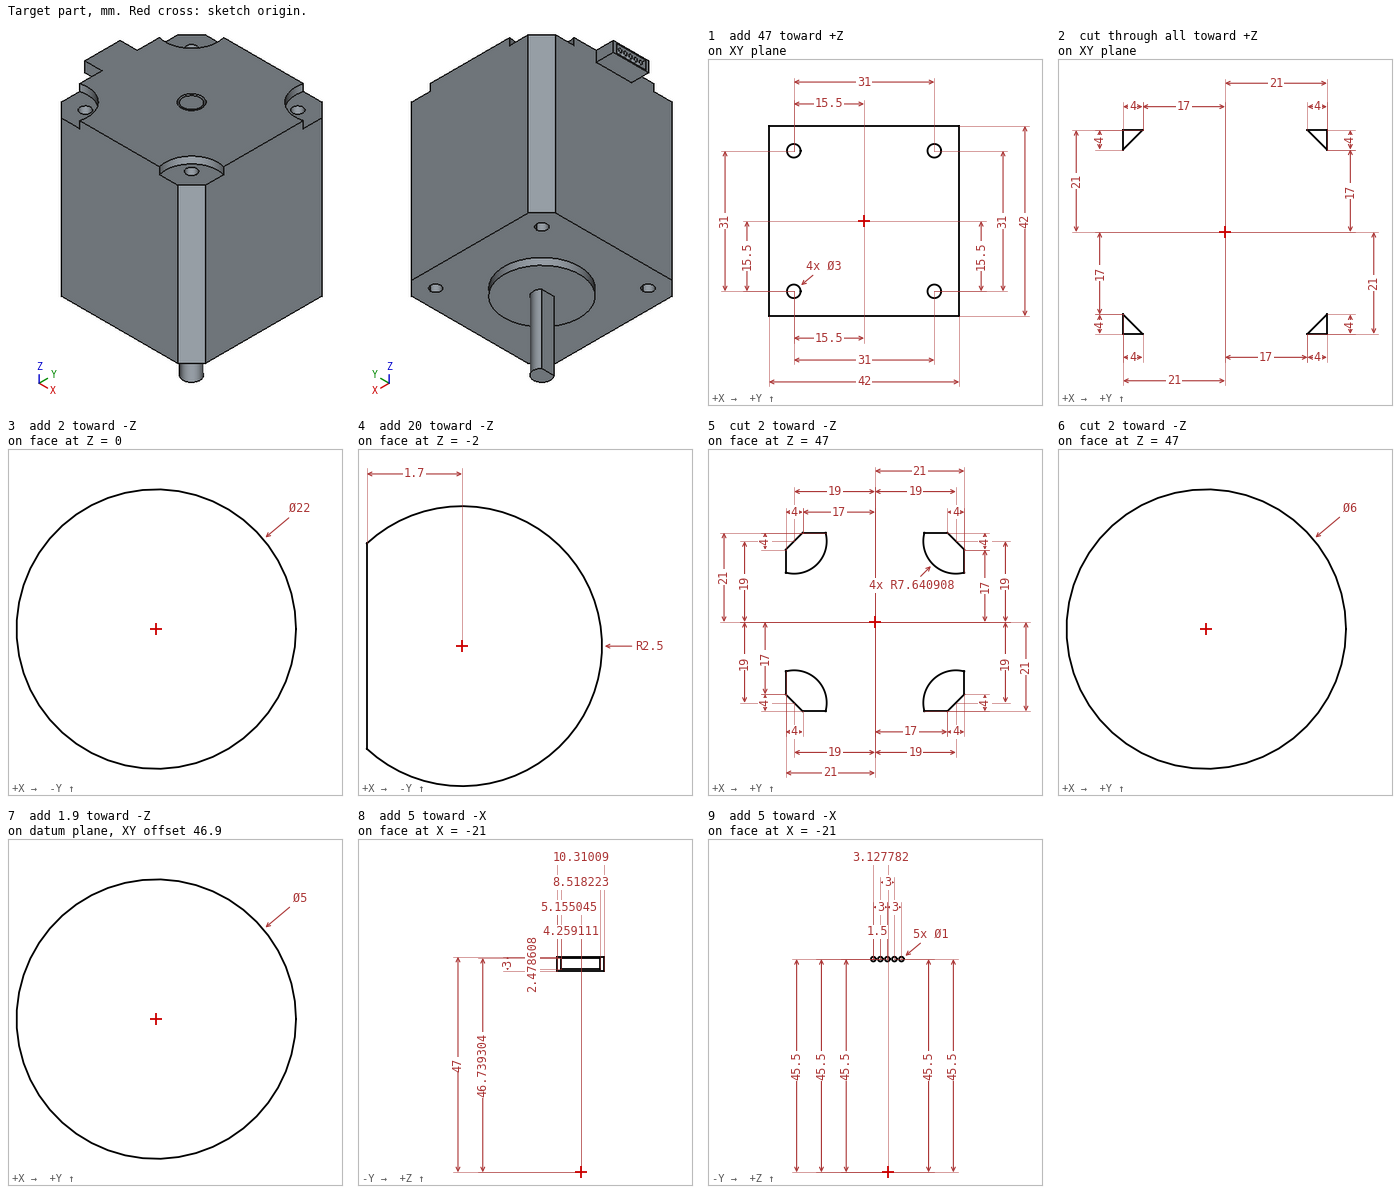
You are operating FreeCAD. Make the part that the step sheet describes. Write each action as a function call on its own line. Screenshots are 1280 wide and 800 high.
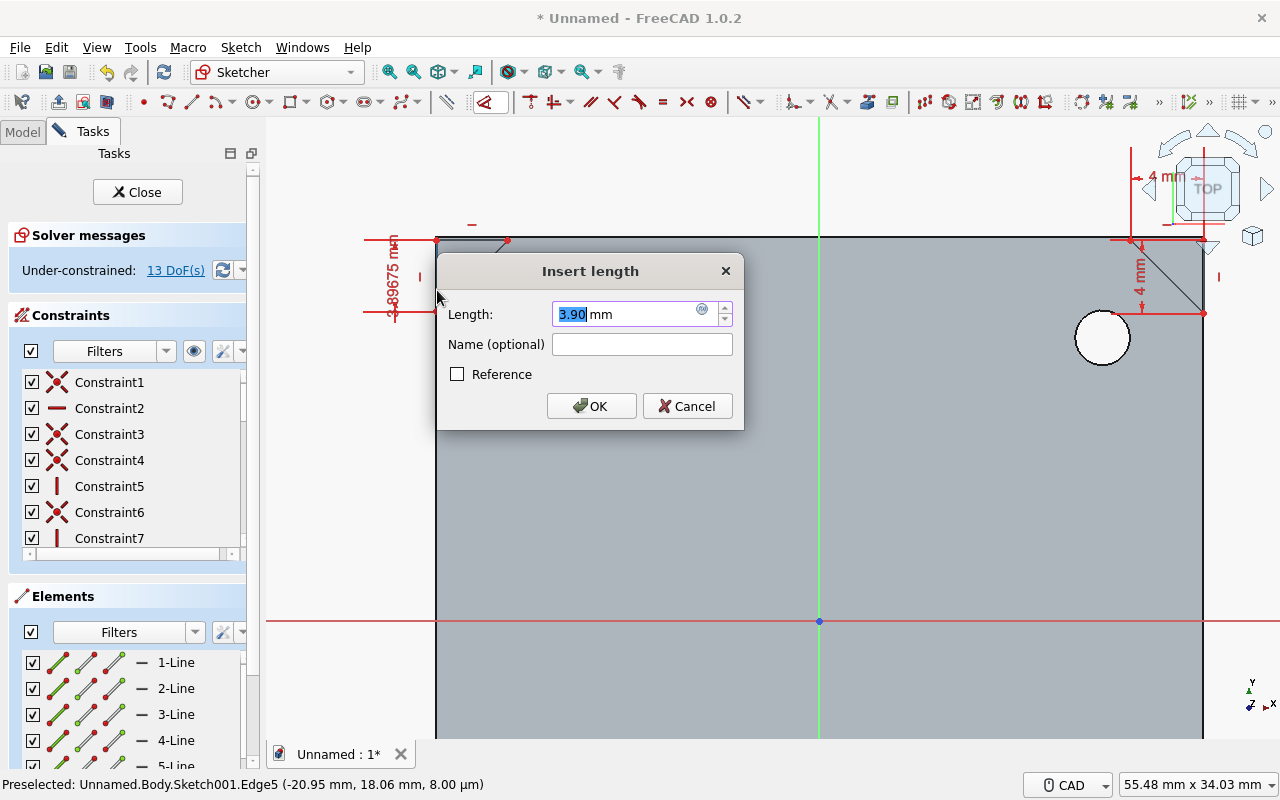
text(4)
key(Return)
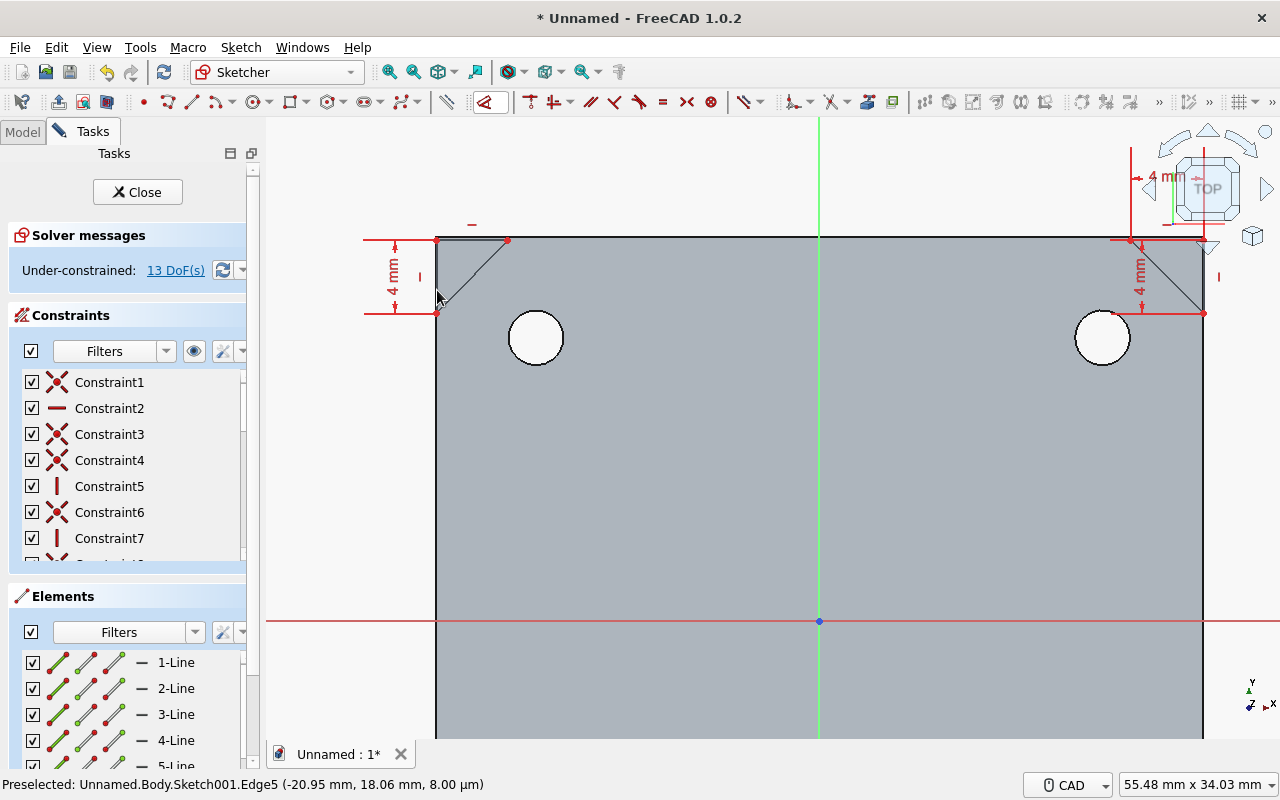
click(458, 240)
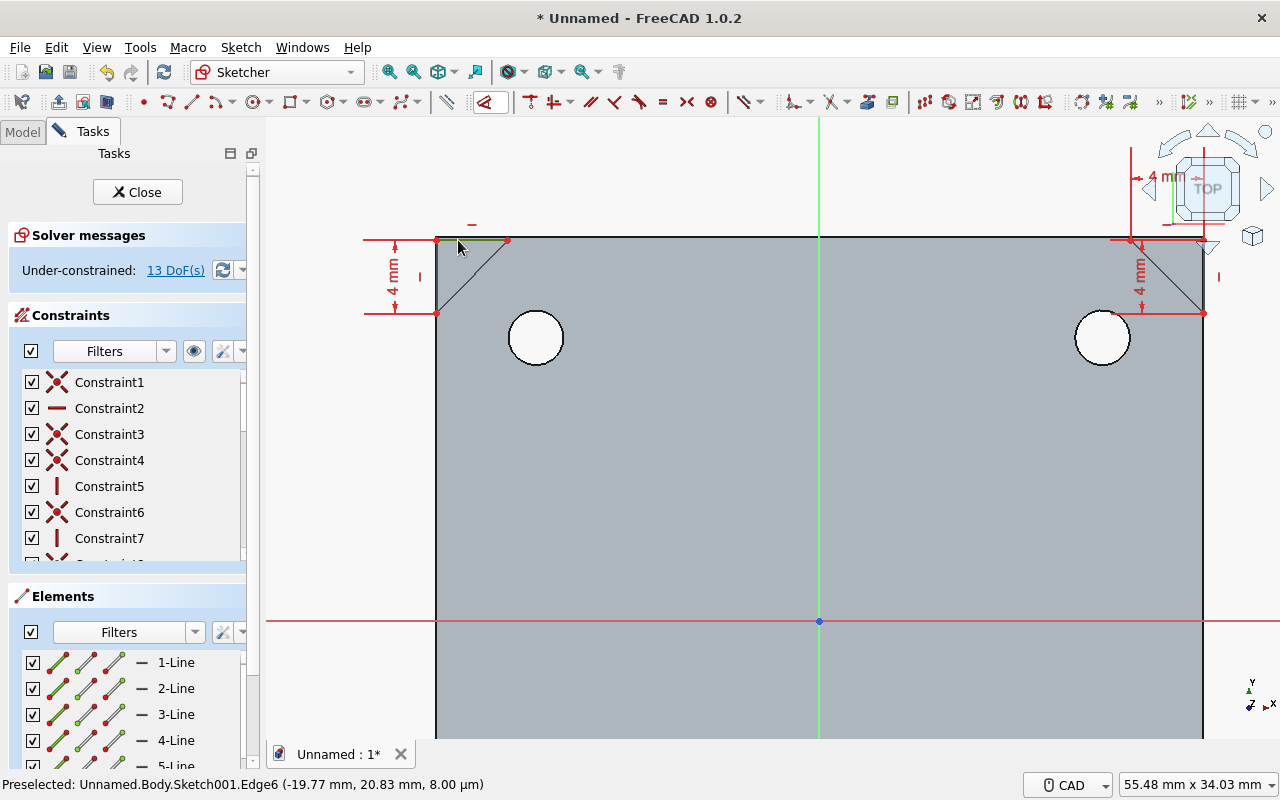
key(l)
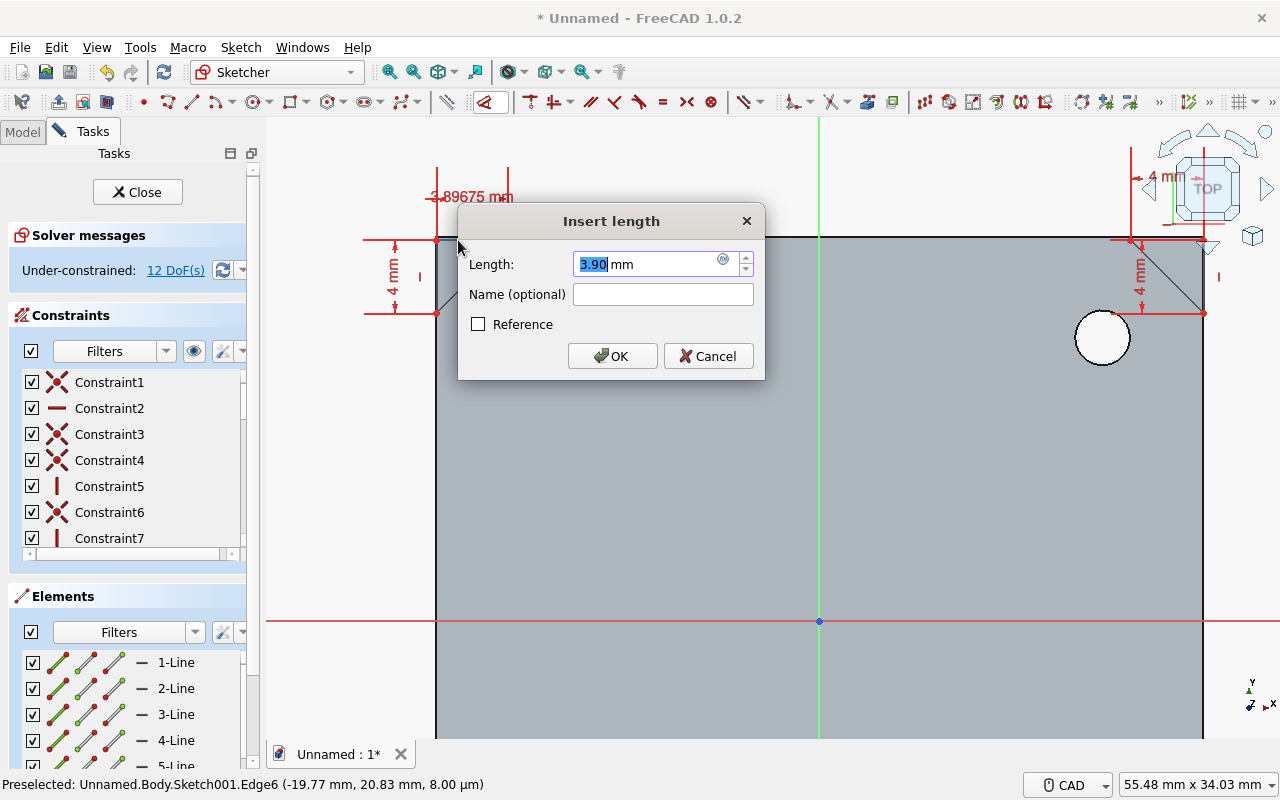
text(4)
key(Return)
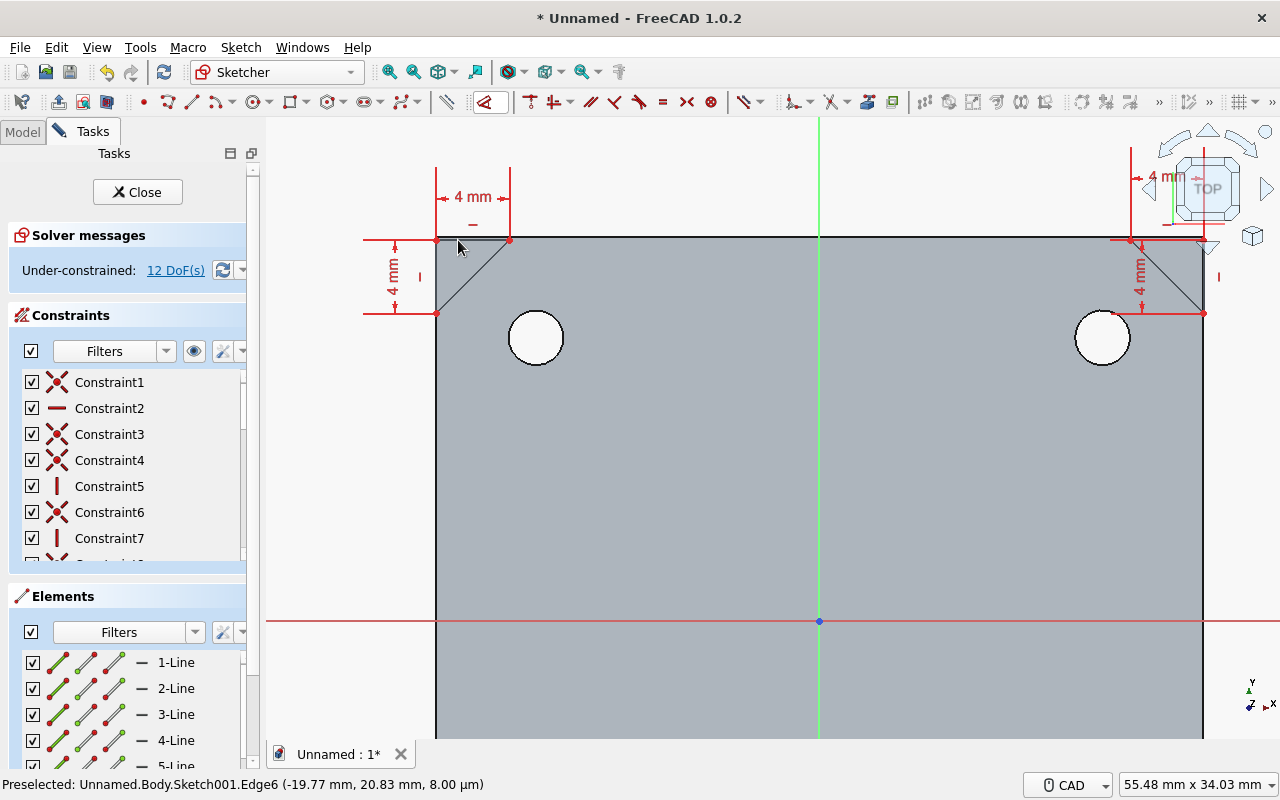
scroll(565, 193, down, 3)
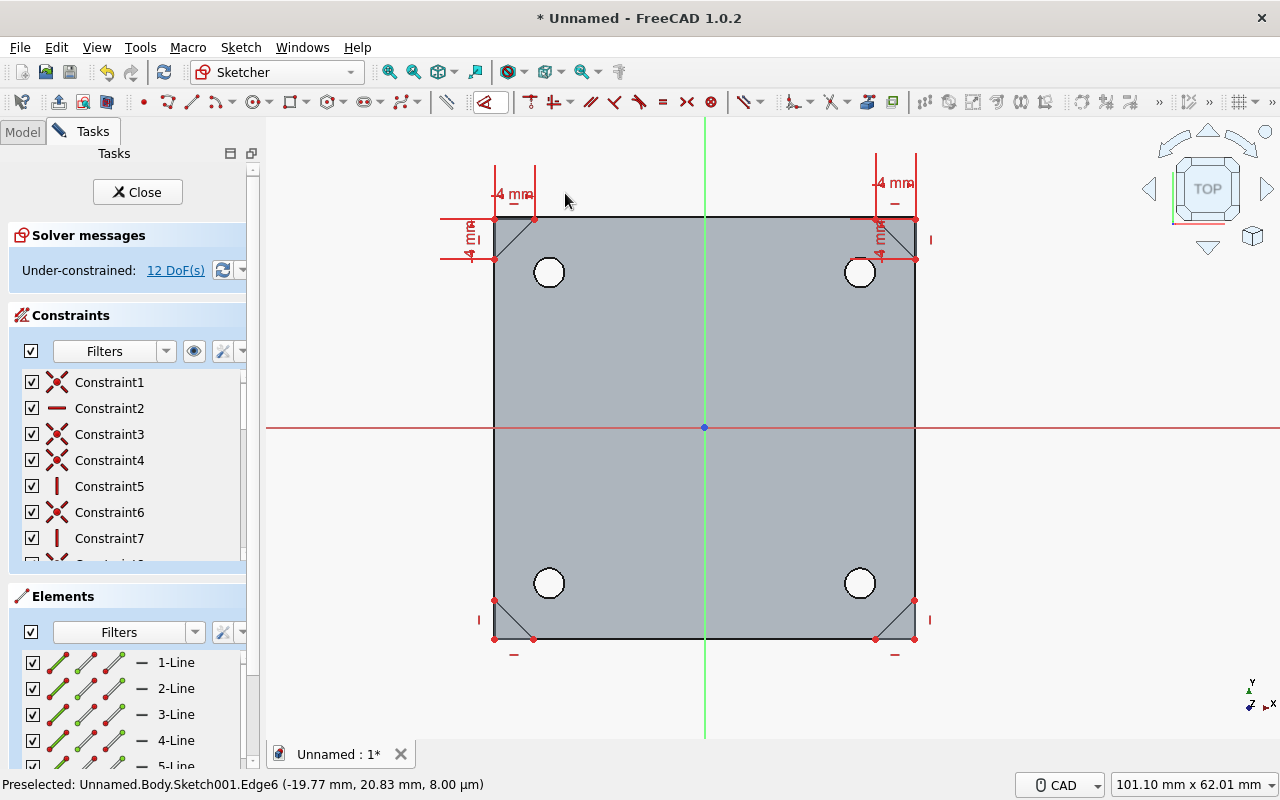
scroll(522, 639, up, 3)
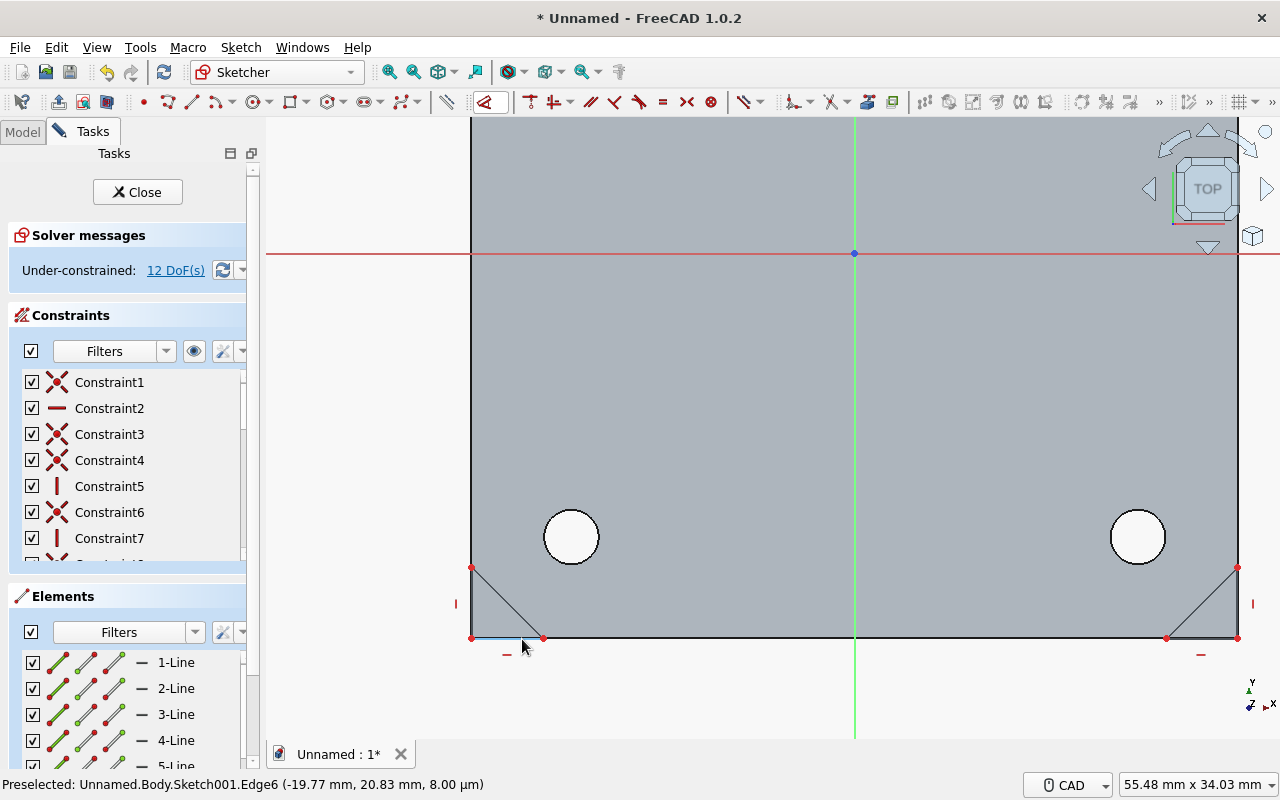
click(522, 639)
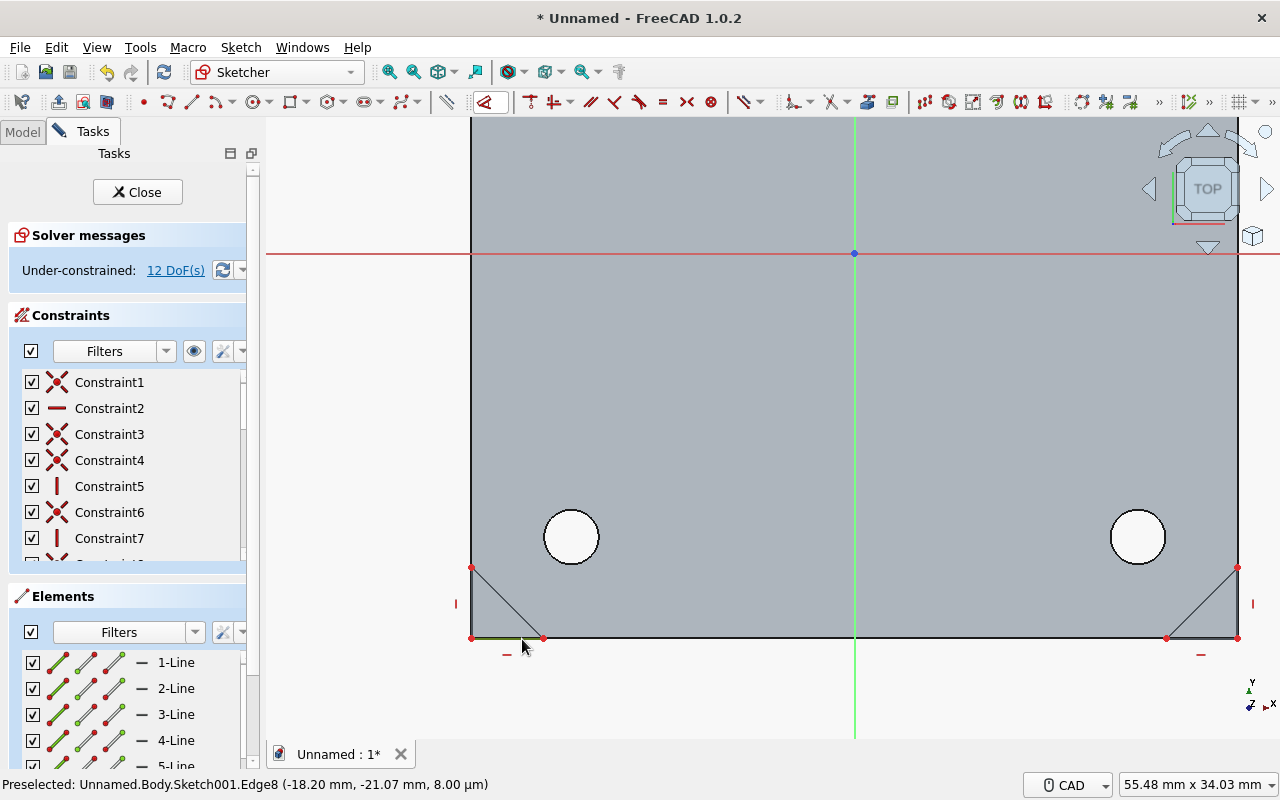
key(l)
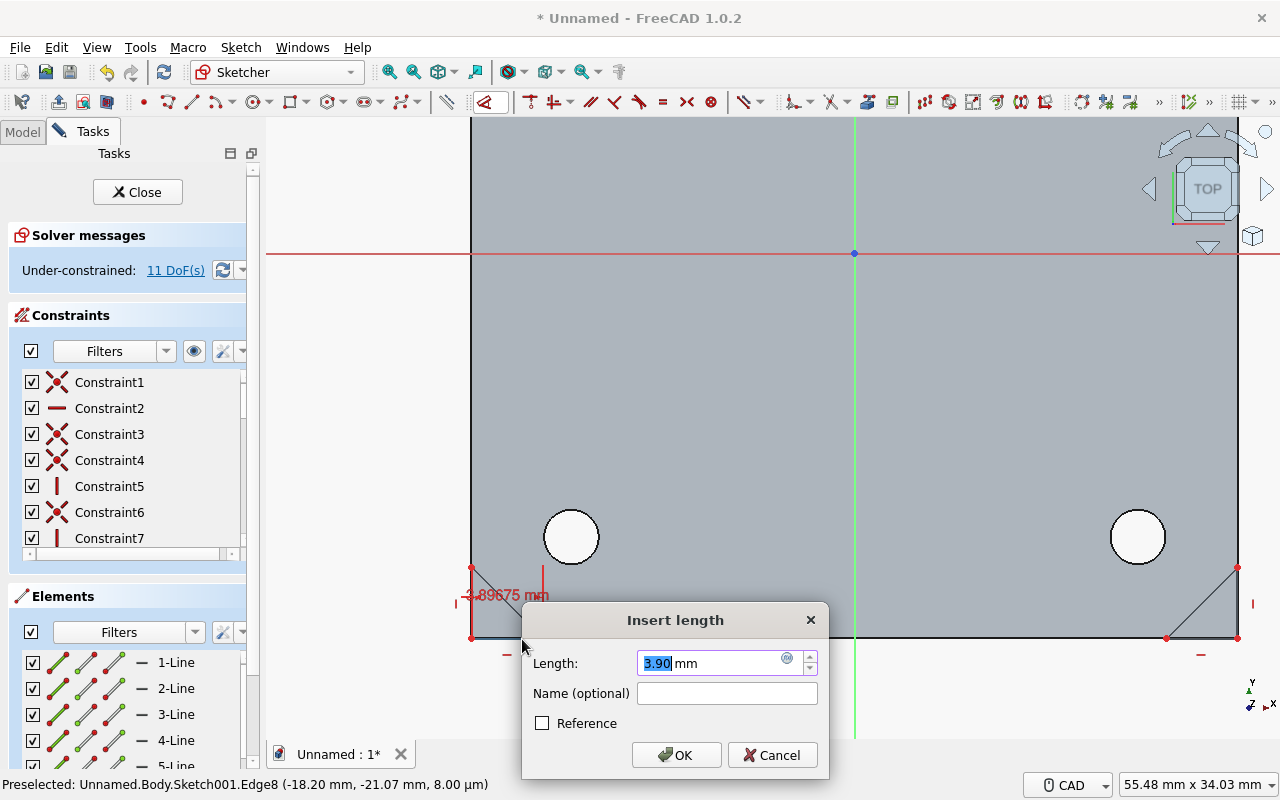
text(4)
key(Return)